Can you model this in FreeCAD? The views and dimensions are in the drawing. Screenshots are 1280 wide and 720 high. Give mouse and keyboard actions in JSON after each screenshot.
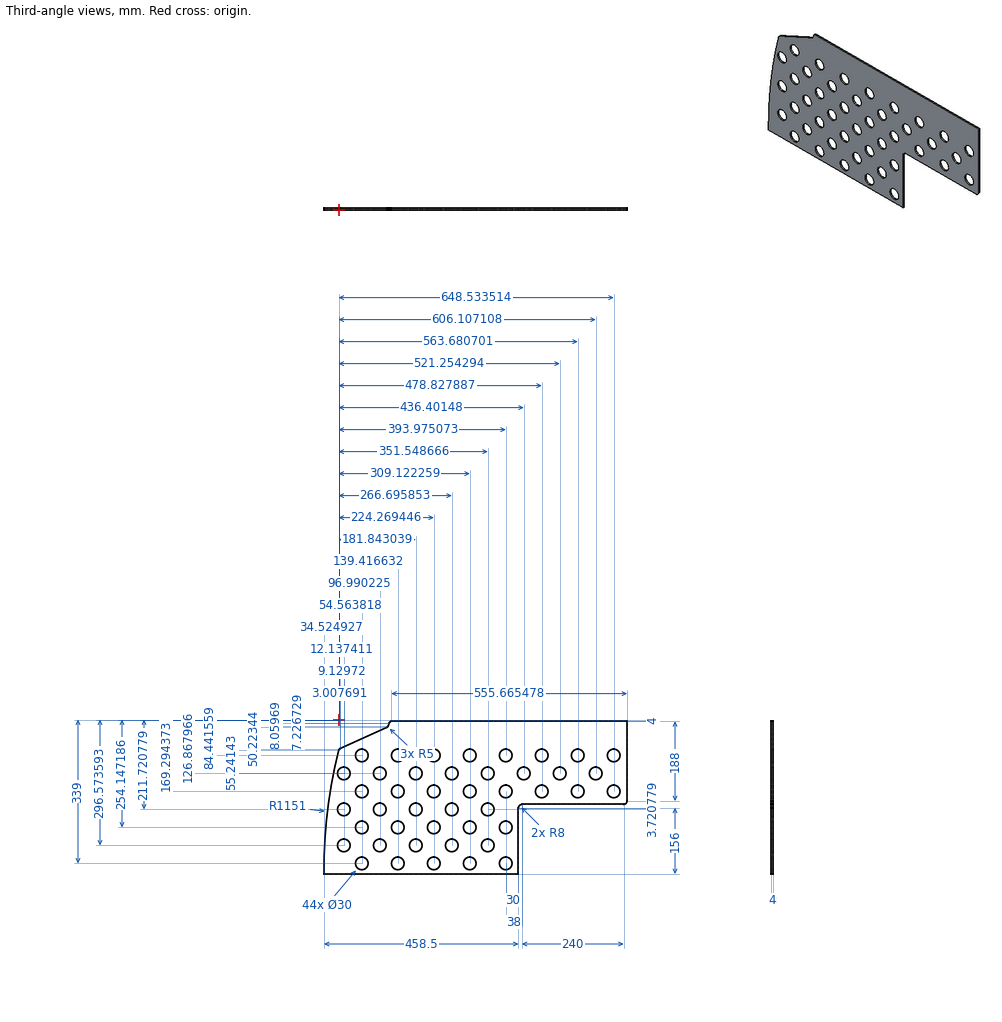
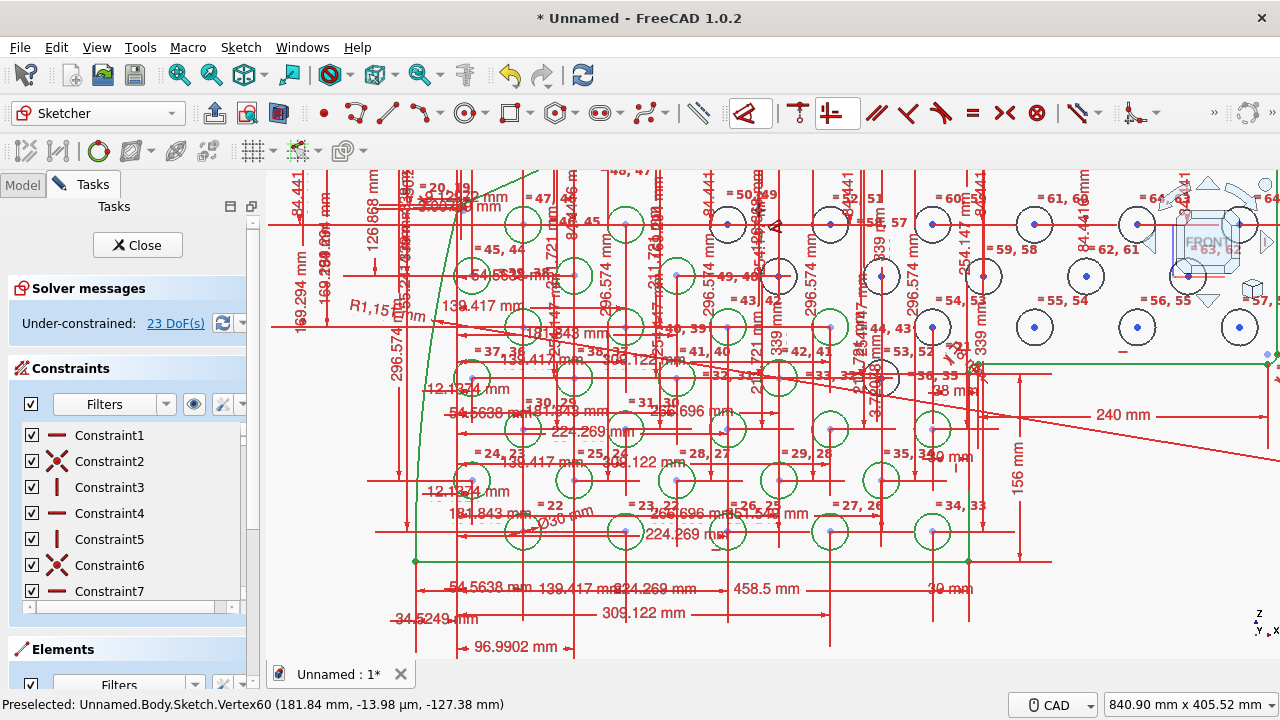
{"action": "left_click", "coordinate": [779, 277]}
{"action": "left_click", "coordinate": [618, 383]}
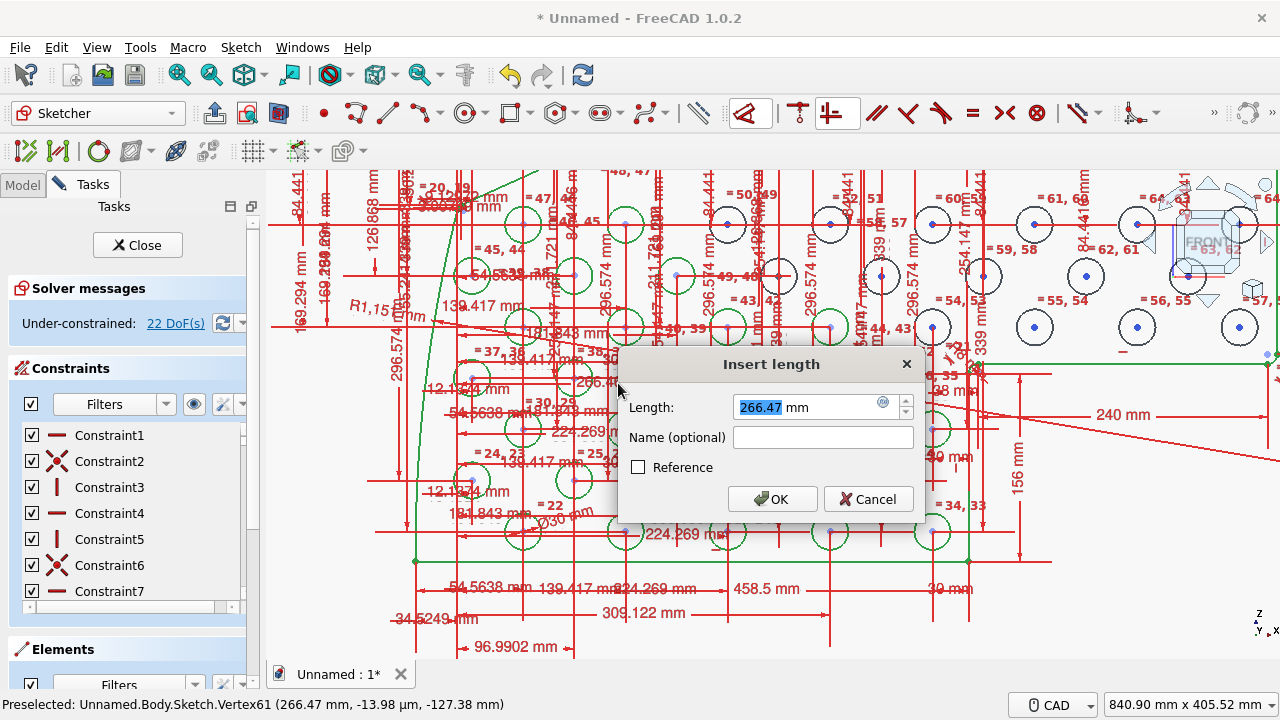
{"action": "type", "text": "266.695853"}
{"action": "key", "text": "Return"}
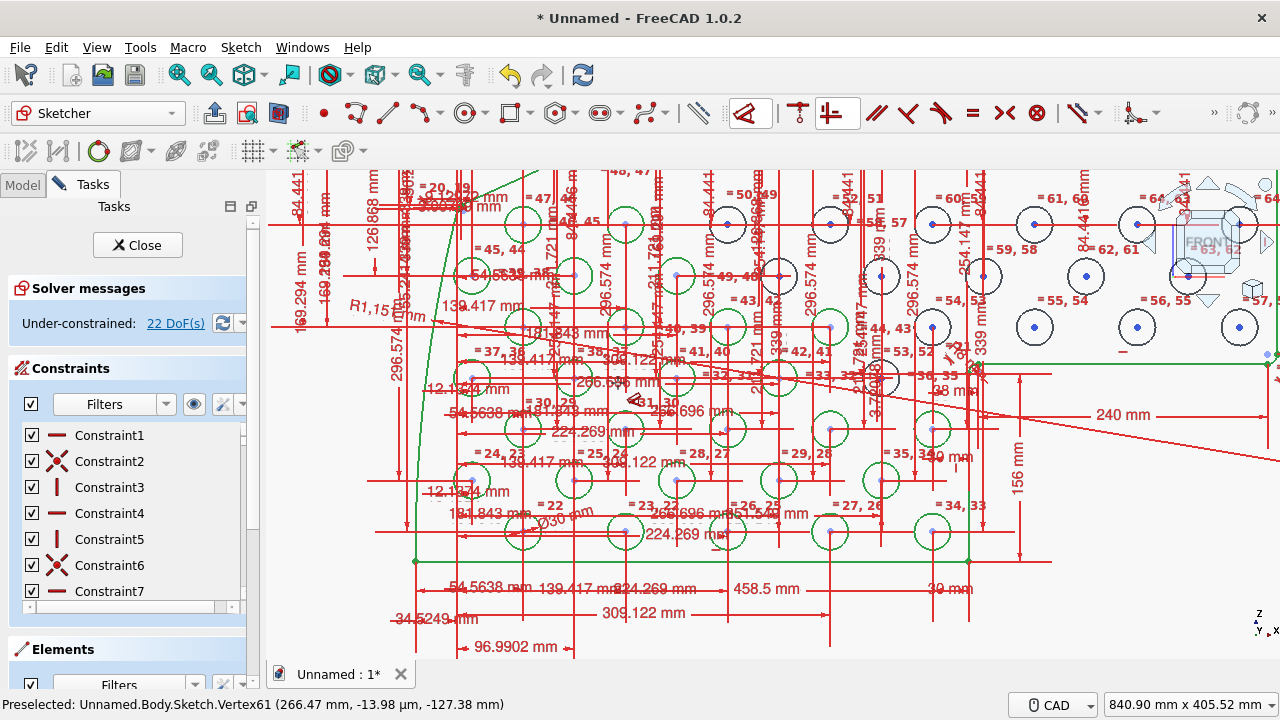
{"action": "left_click", "coordinate": [779, 277]}
{"action": "left_click", "coordinate": [861, 210]}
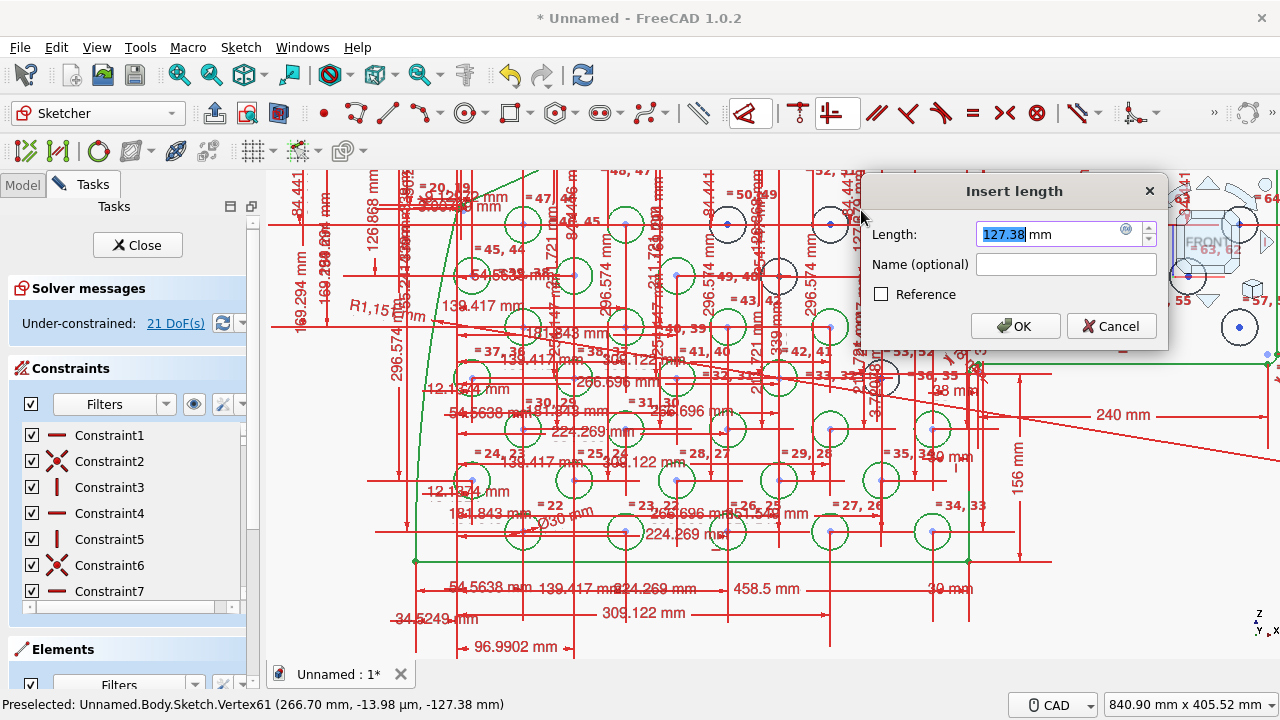
{"action": "type", "text": "126.867966"}
{"action": "key", "text": "Return"}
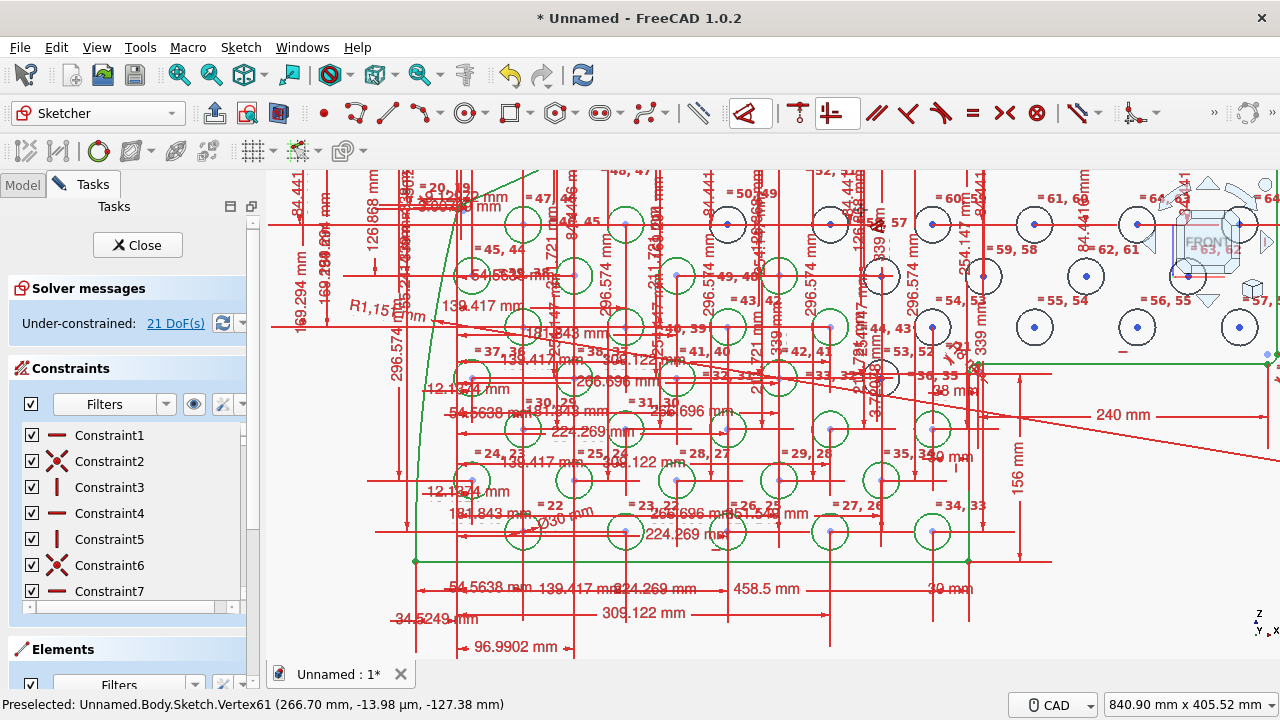
{"action": "left_click", "coordinate": [728, 225]}
{"action": "left_click", "coordinate": [593, 259]}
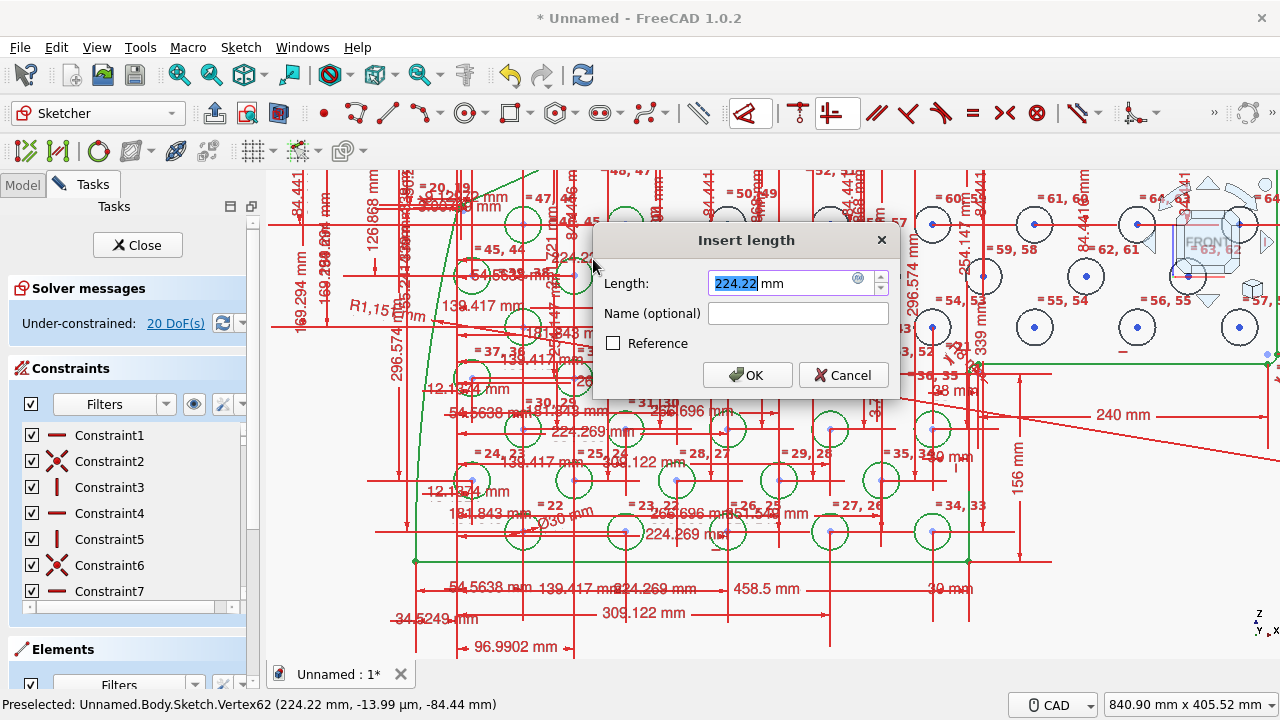
{"action": "type", "text": "224.269446"}
{"action": "key", "text": "Return"}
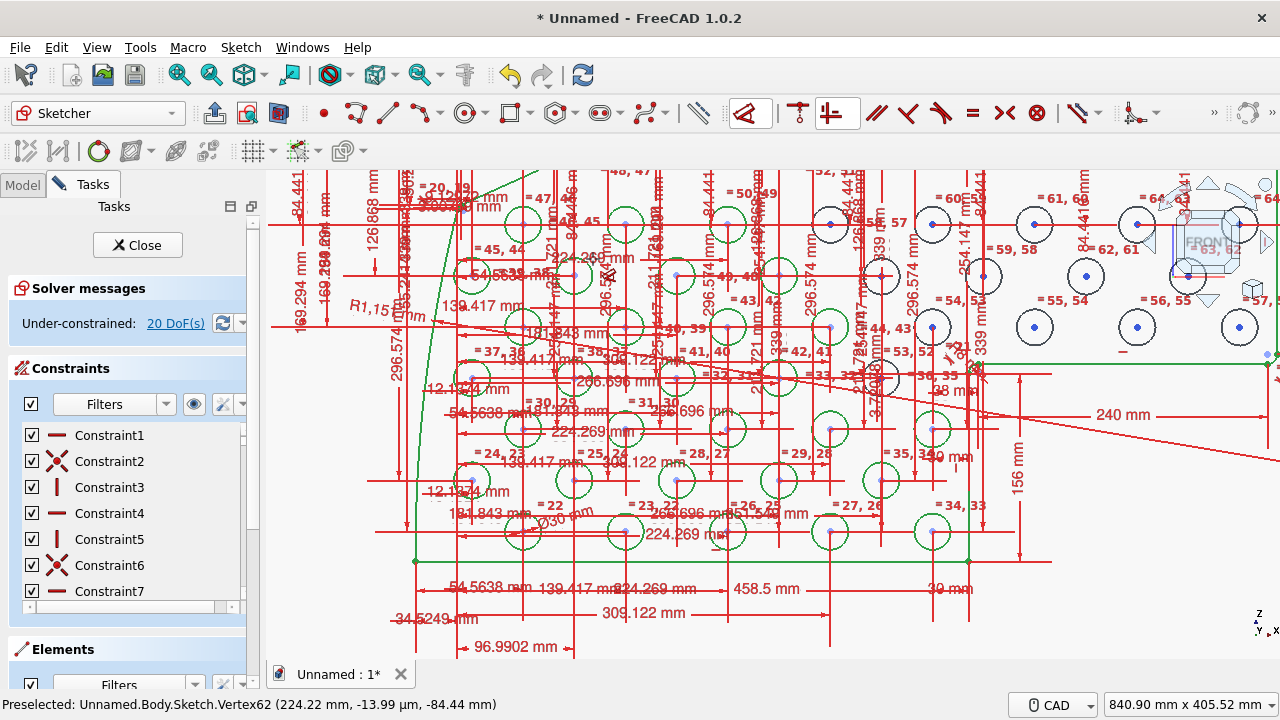
{"action": "left_click", "coordinate": [830, 225]}
{"action": "left_click", "coordinate": [774, 307]}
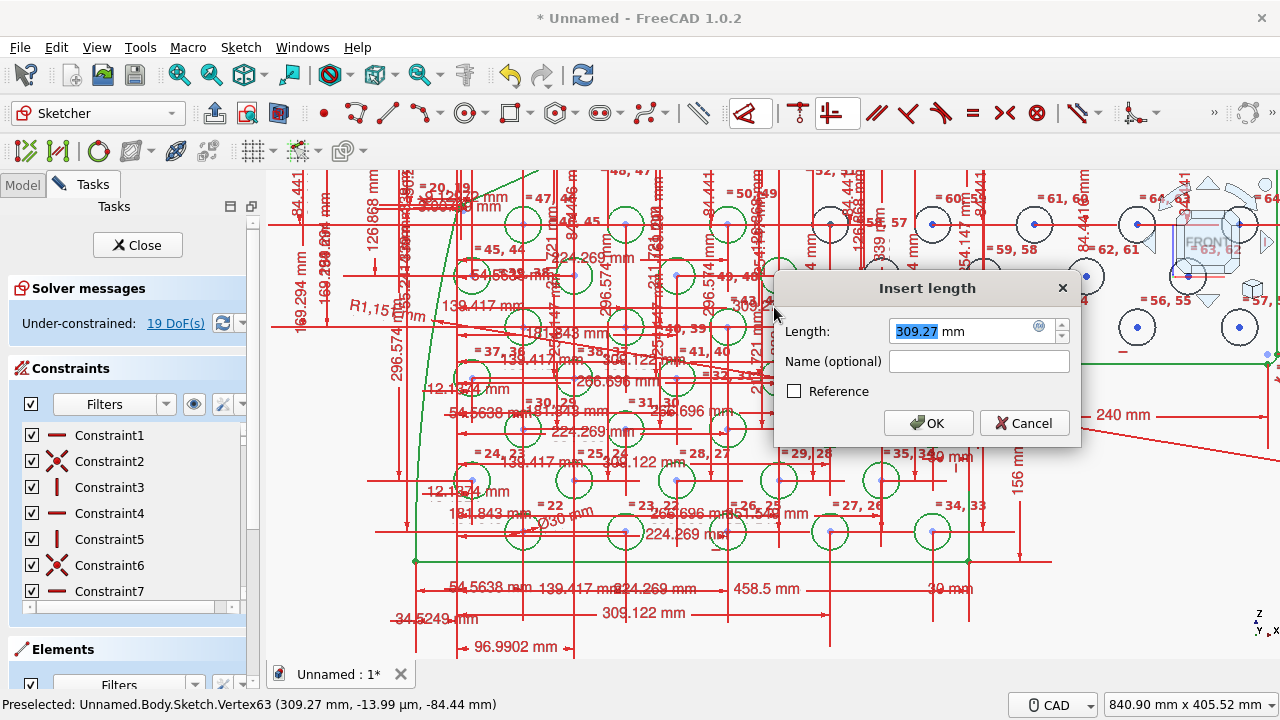
{"action": "type", "text": "309.122259"}
{"action": "key", "text": "Return"}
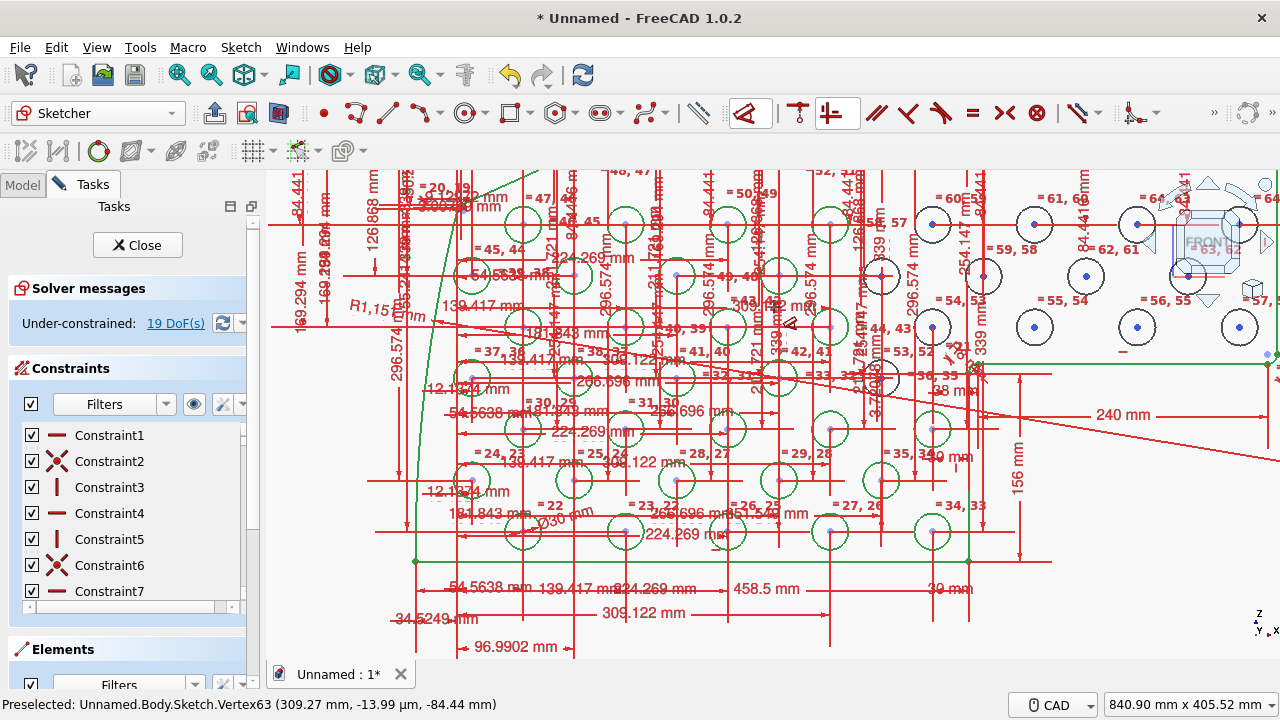
{"action": "left_click", "coordinate": [881, 378]}
{"action": "left_click", "coordinate": [767, 412]}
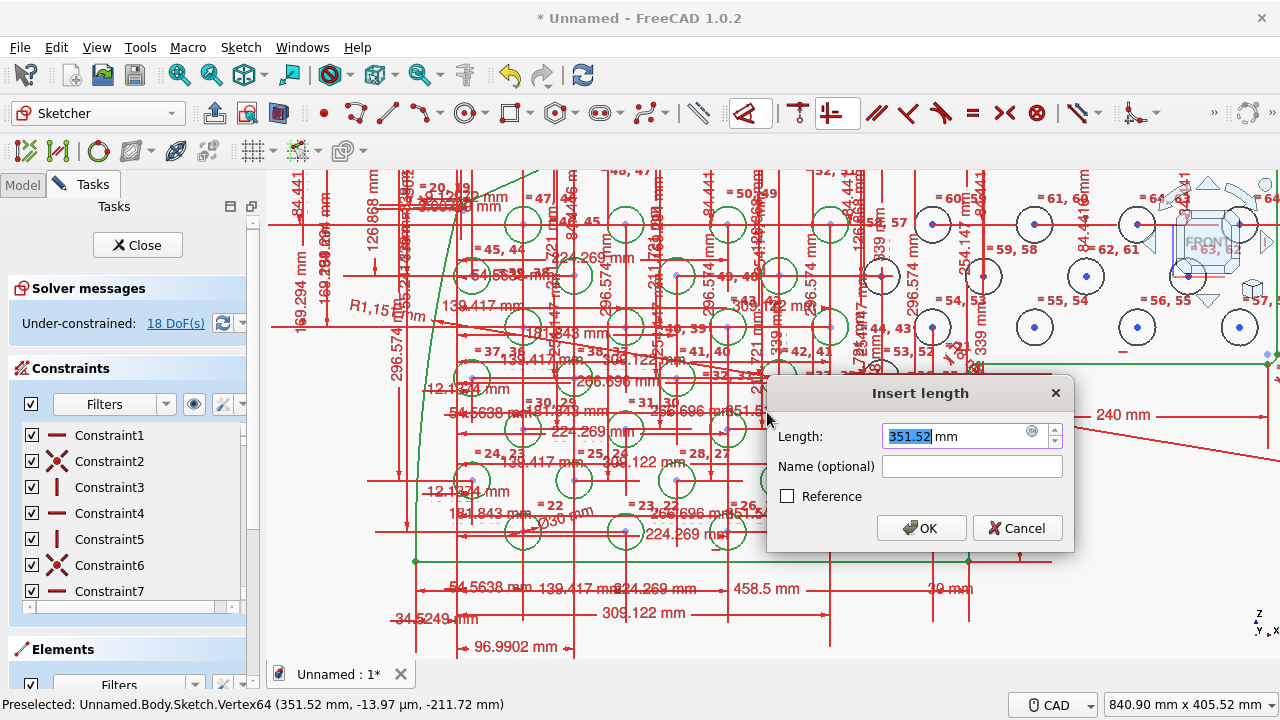
{"action": "type", "text": "351.548666"}
{"action": "key", "text": "Return"}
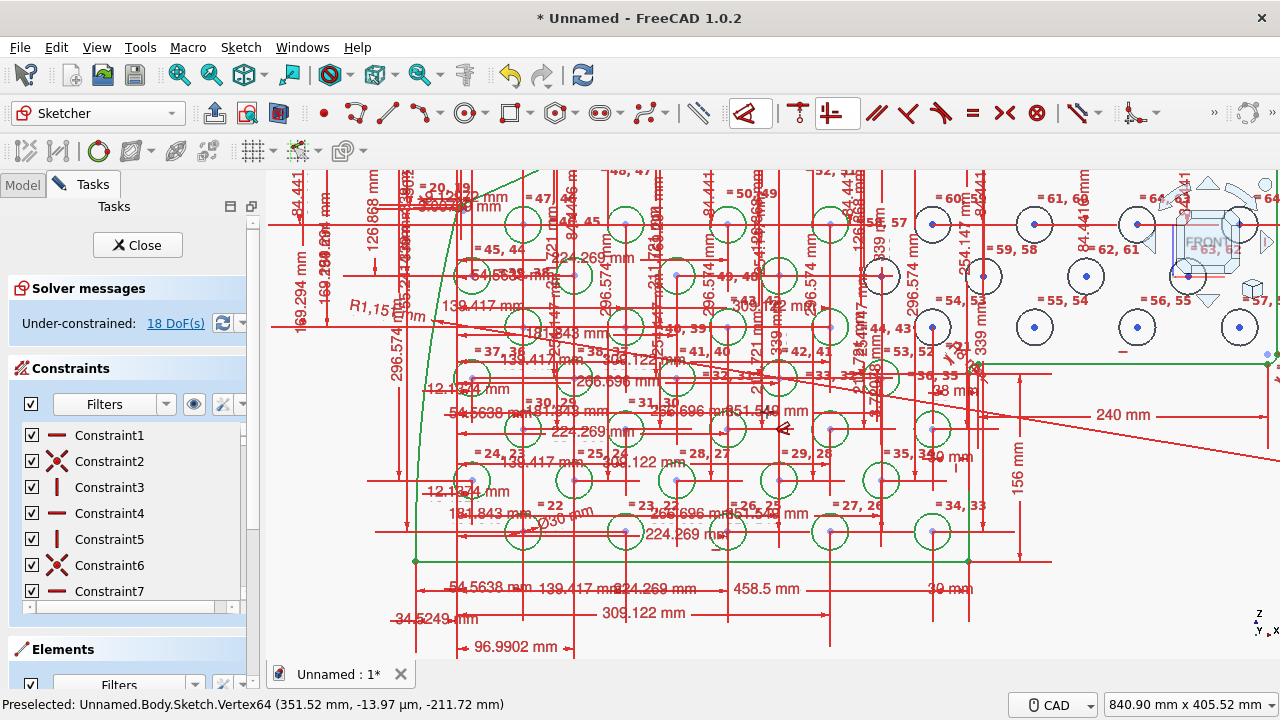
{"action": "left_click", "coordinate": [933, 327]}
{"action": "left_click", "coordinate": [1015, 263]}